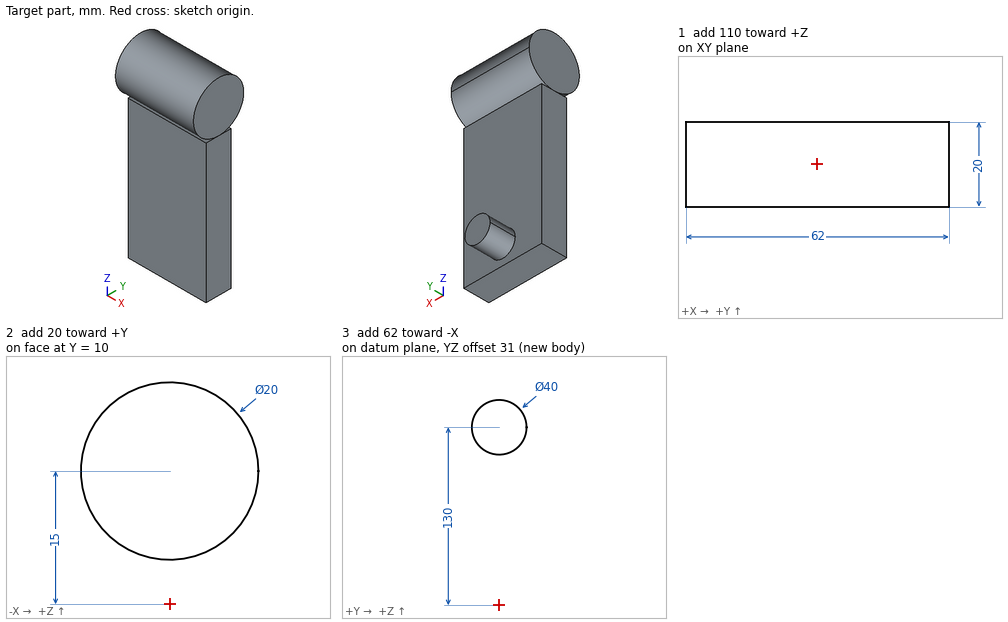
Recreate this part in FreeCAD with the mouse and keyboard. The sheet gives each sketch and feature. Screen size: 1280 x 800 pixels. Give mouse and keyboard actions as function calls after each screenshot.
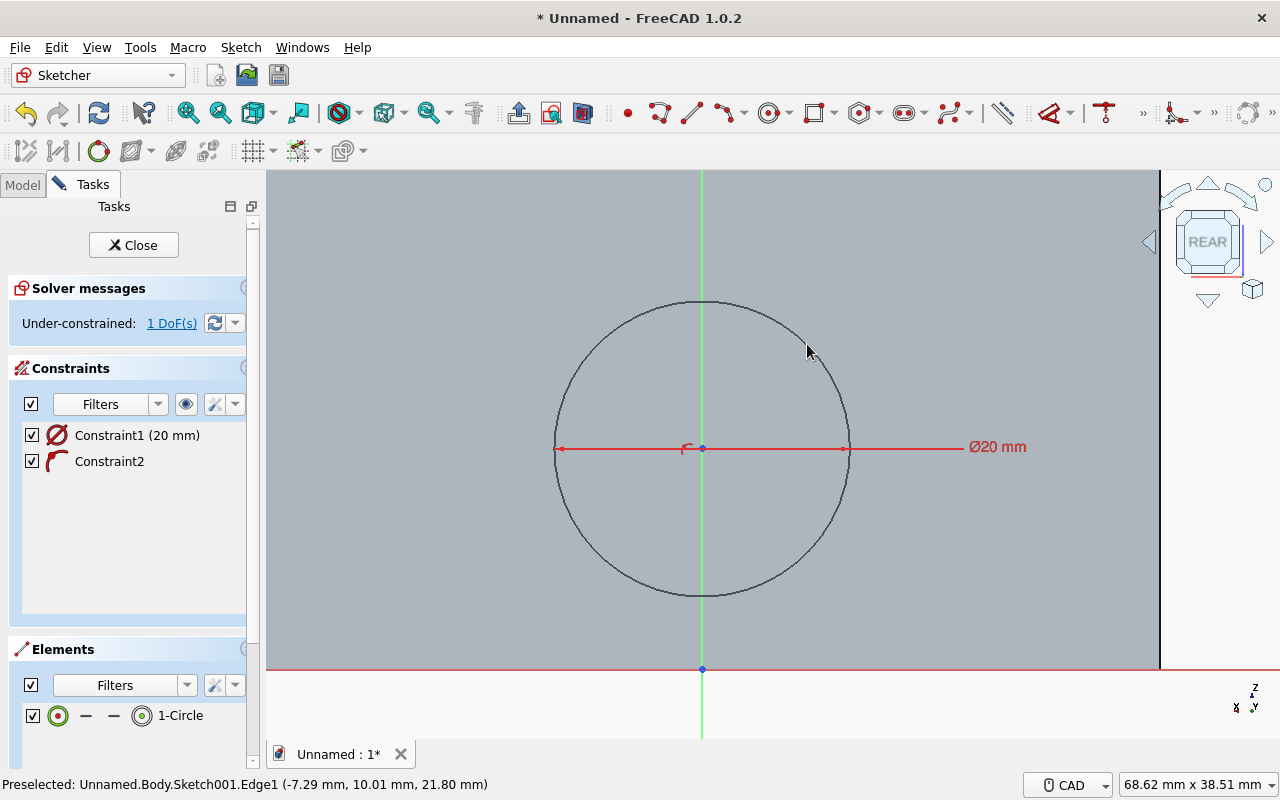
key(d)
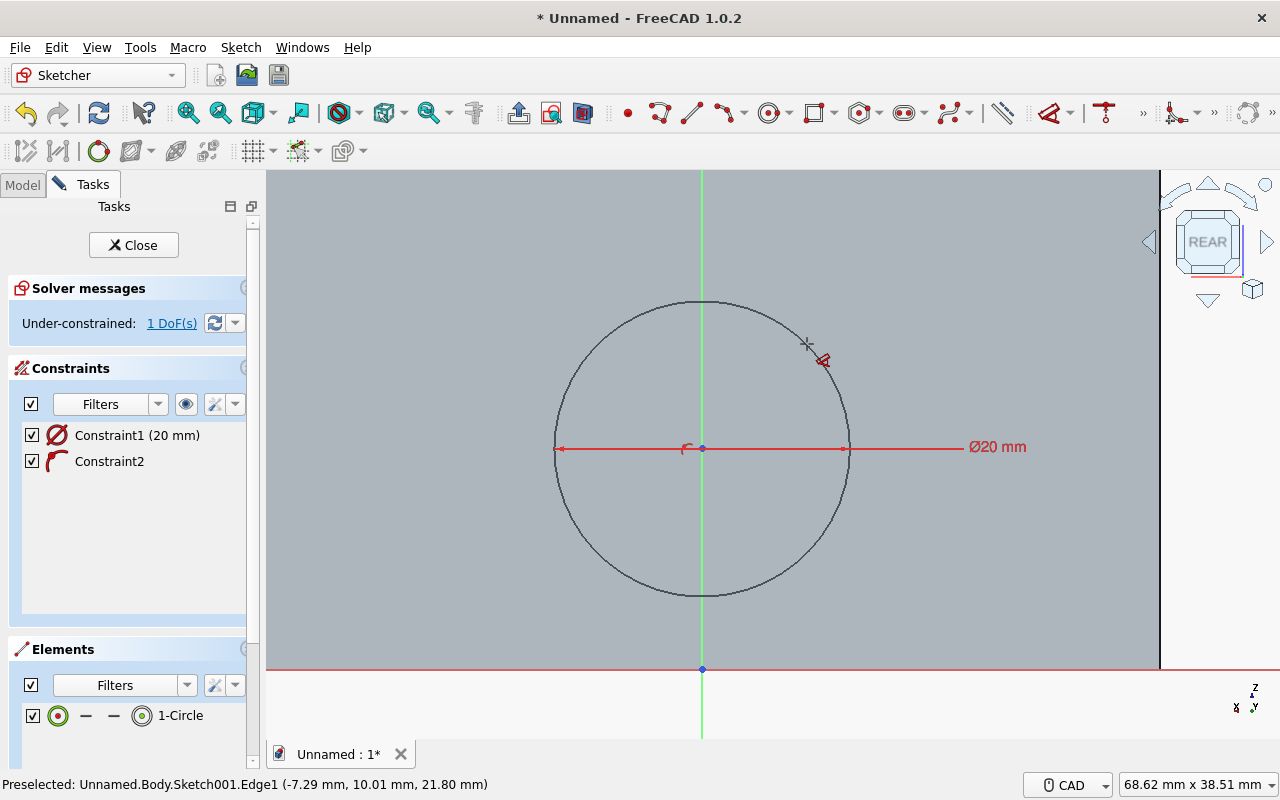
click(702, 449)
click(736, 559)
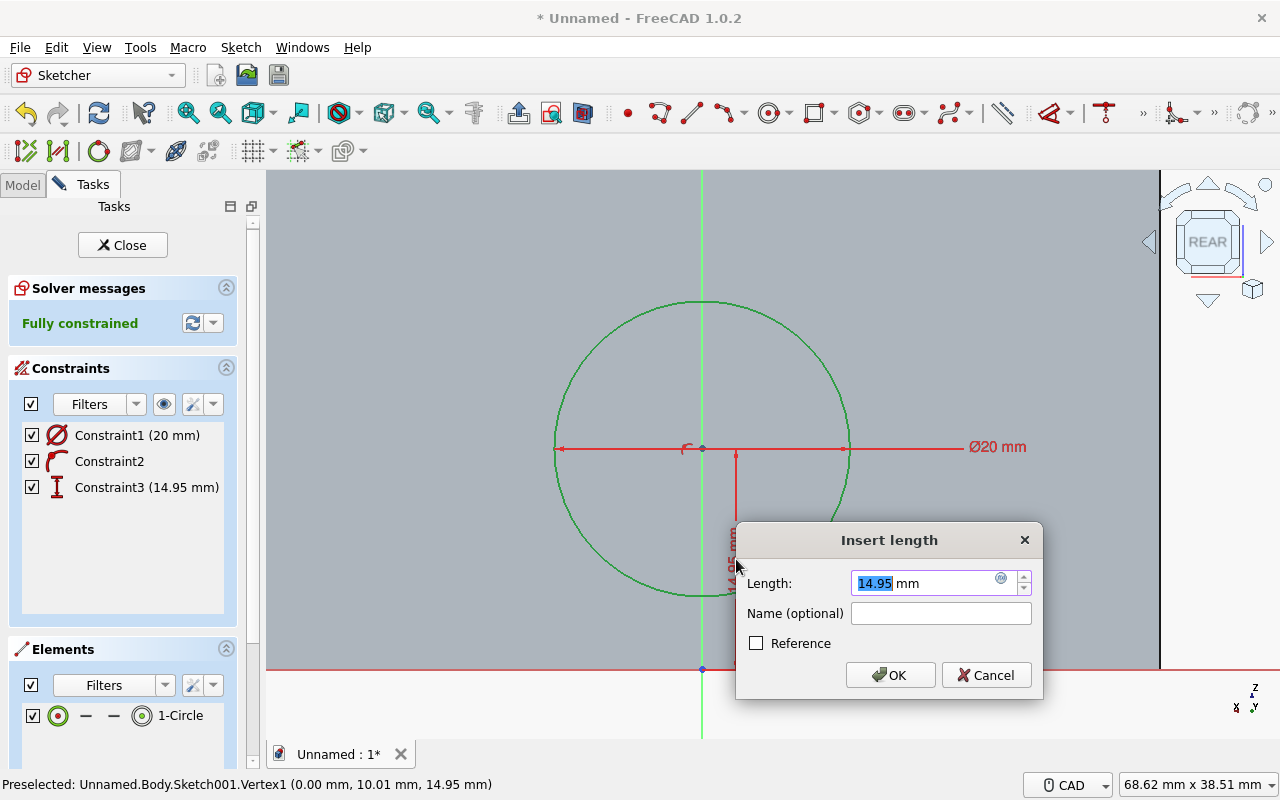
text(15)
key(Return)
key(Escape)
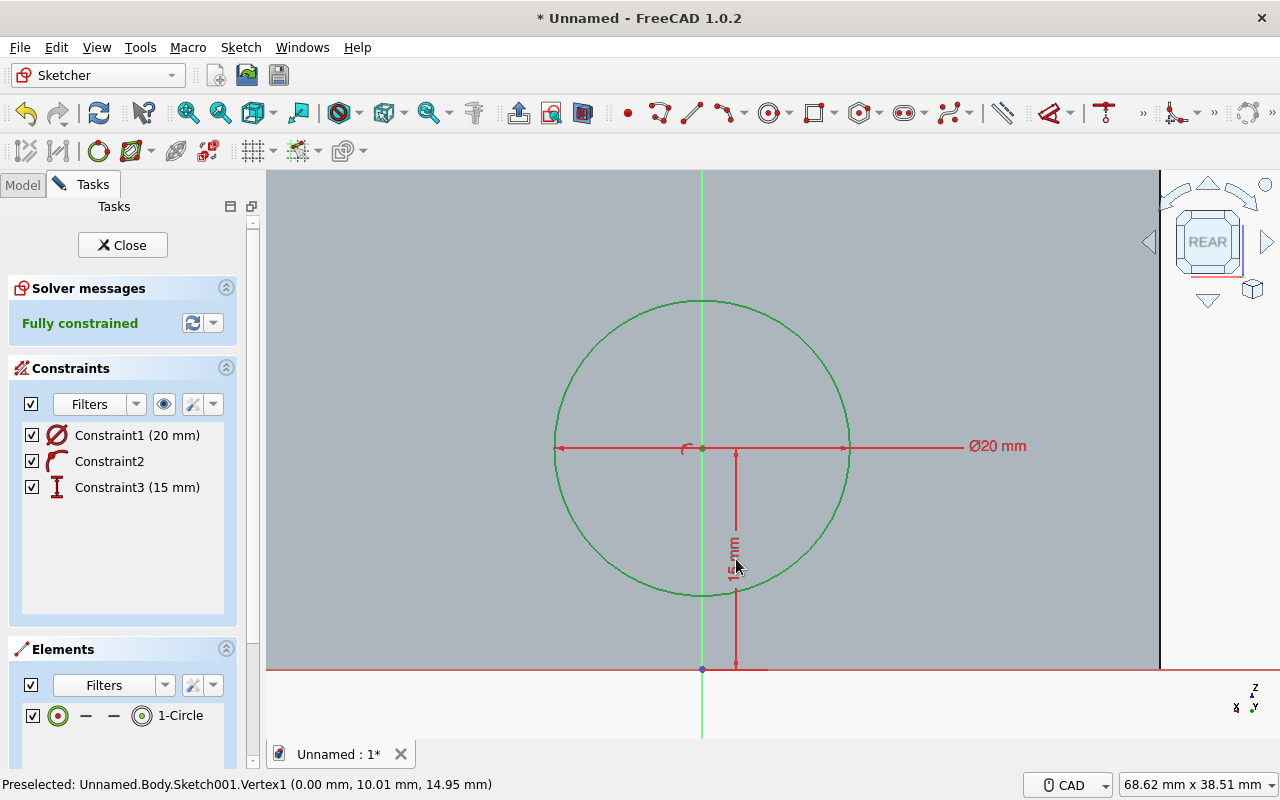
click(123, 245)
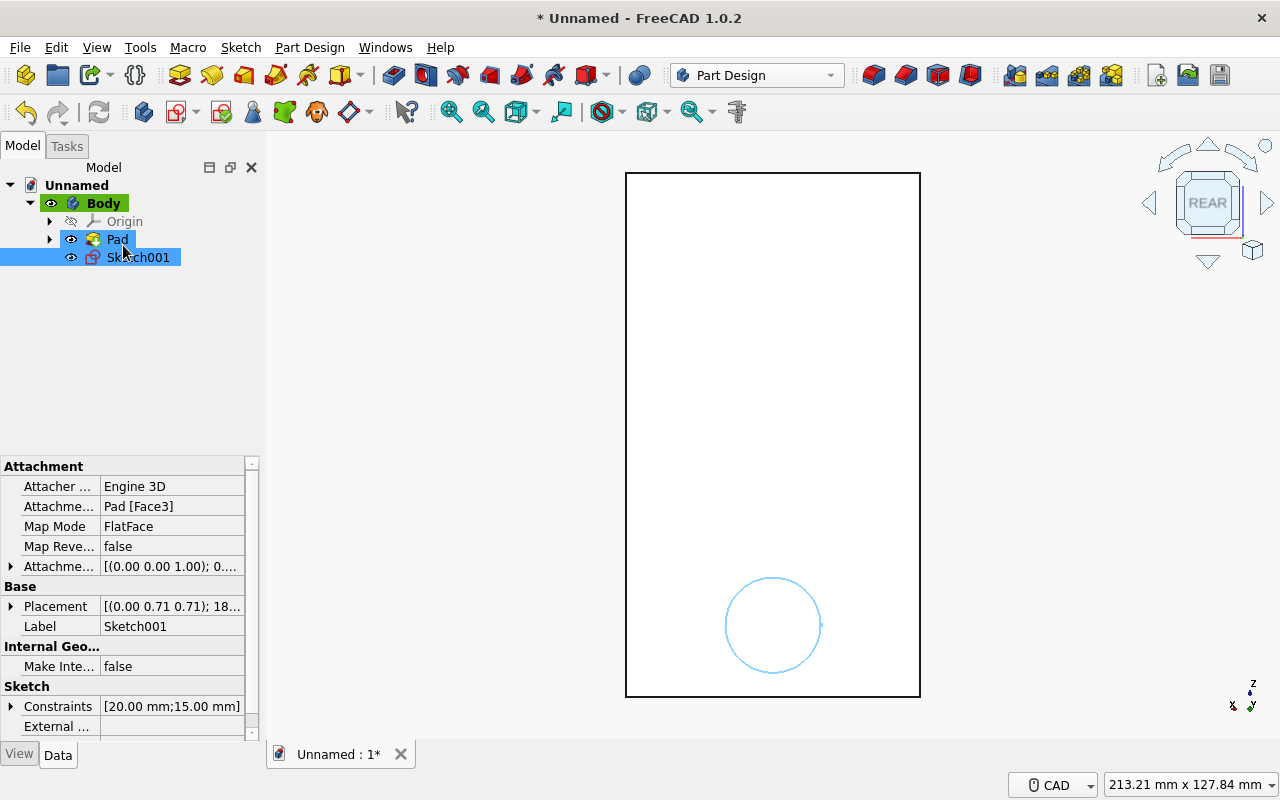
click(180, 76)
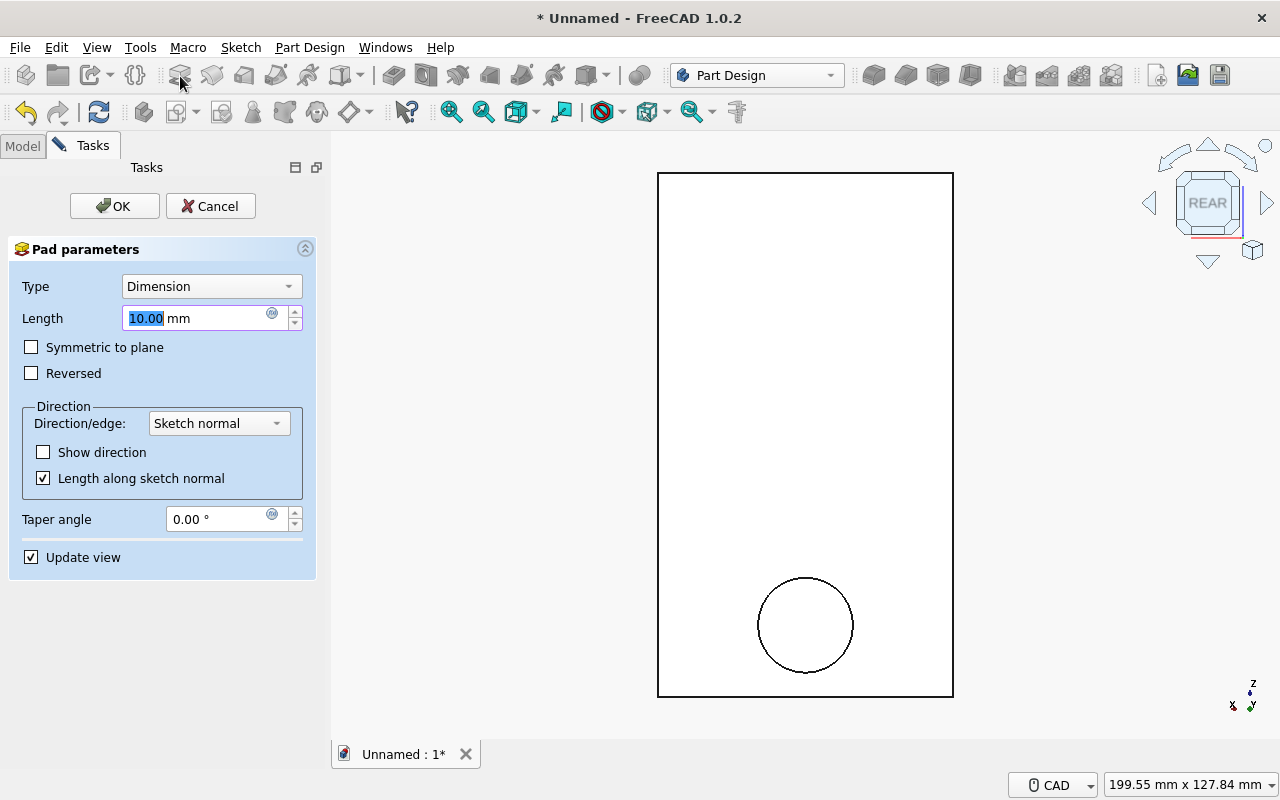
text(20)
key(Tab)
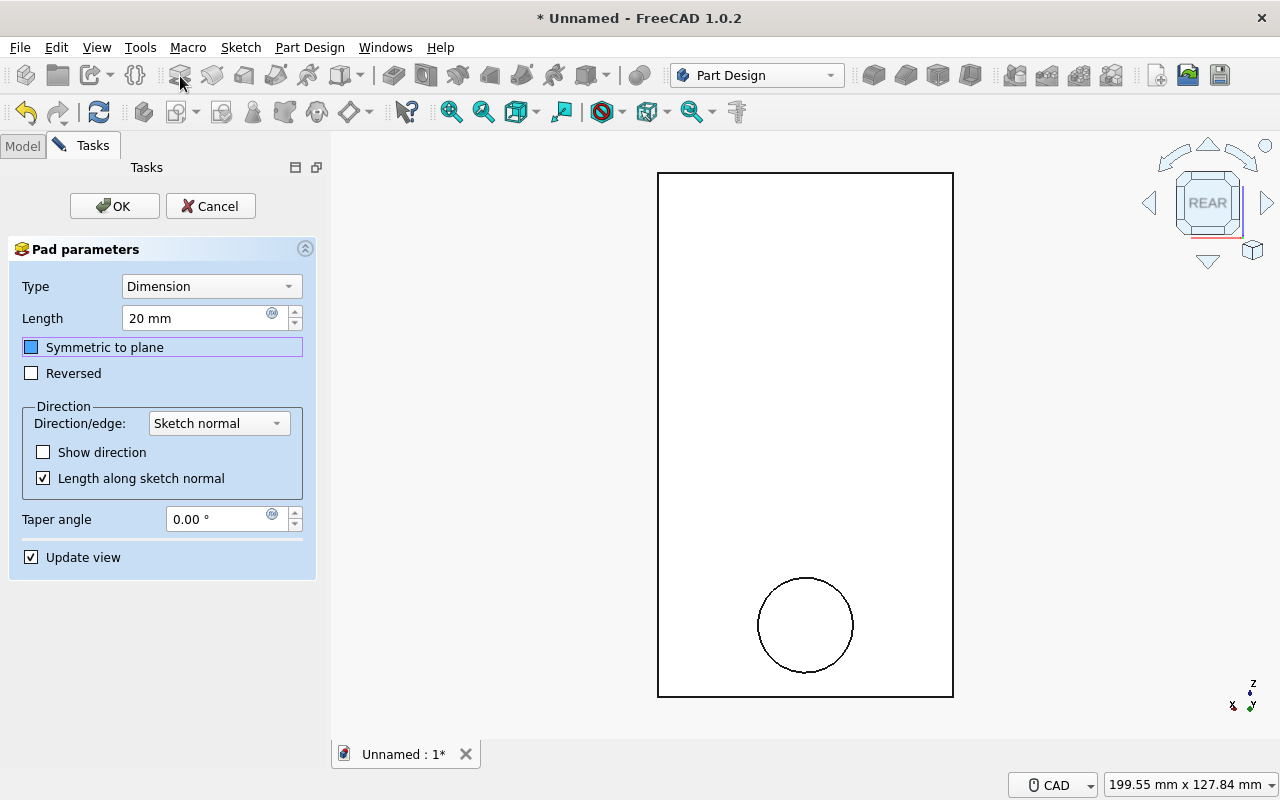
click(115, 206)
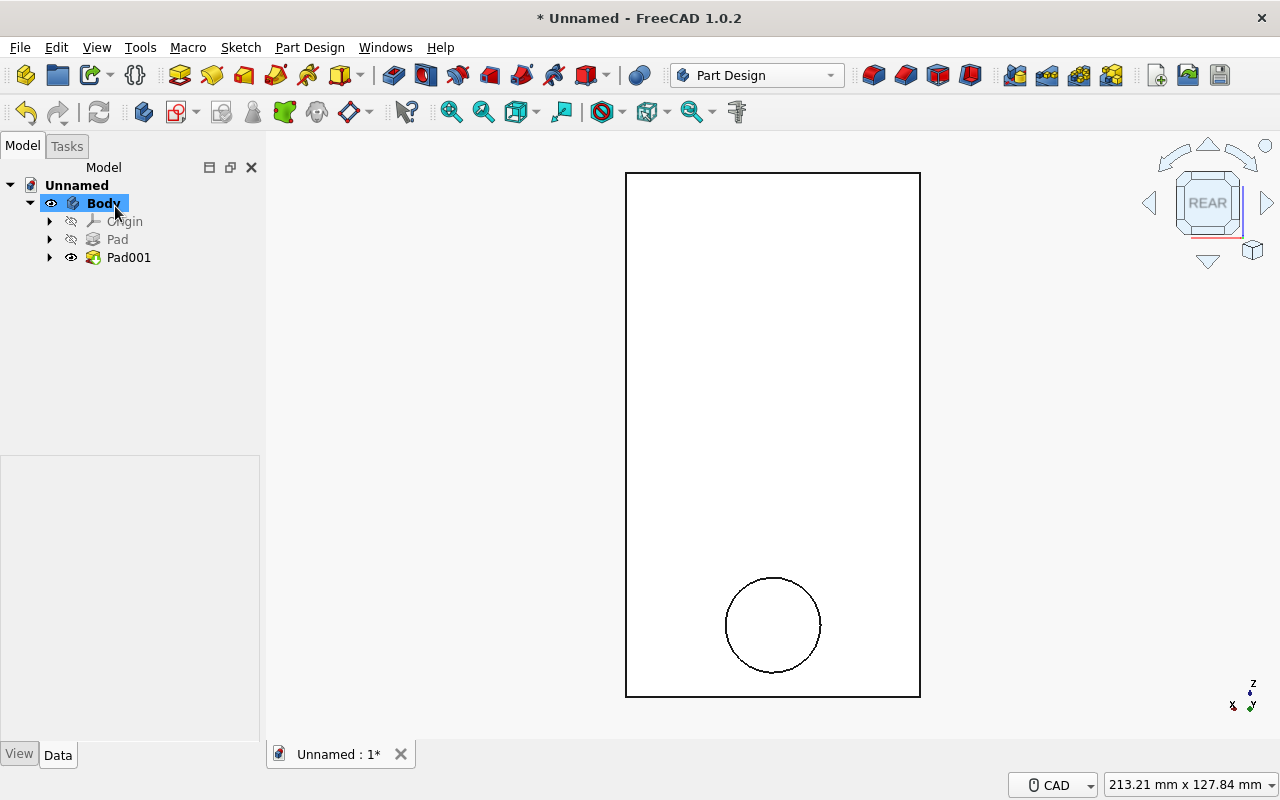
click(144, 112)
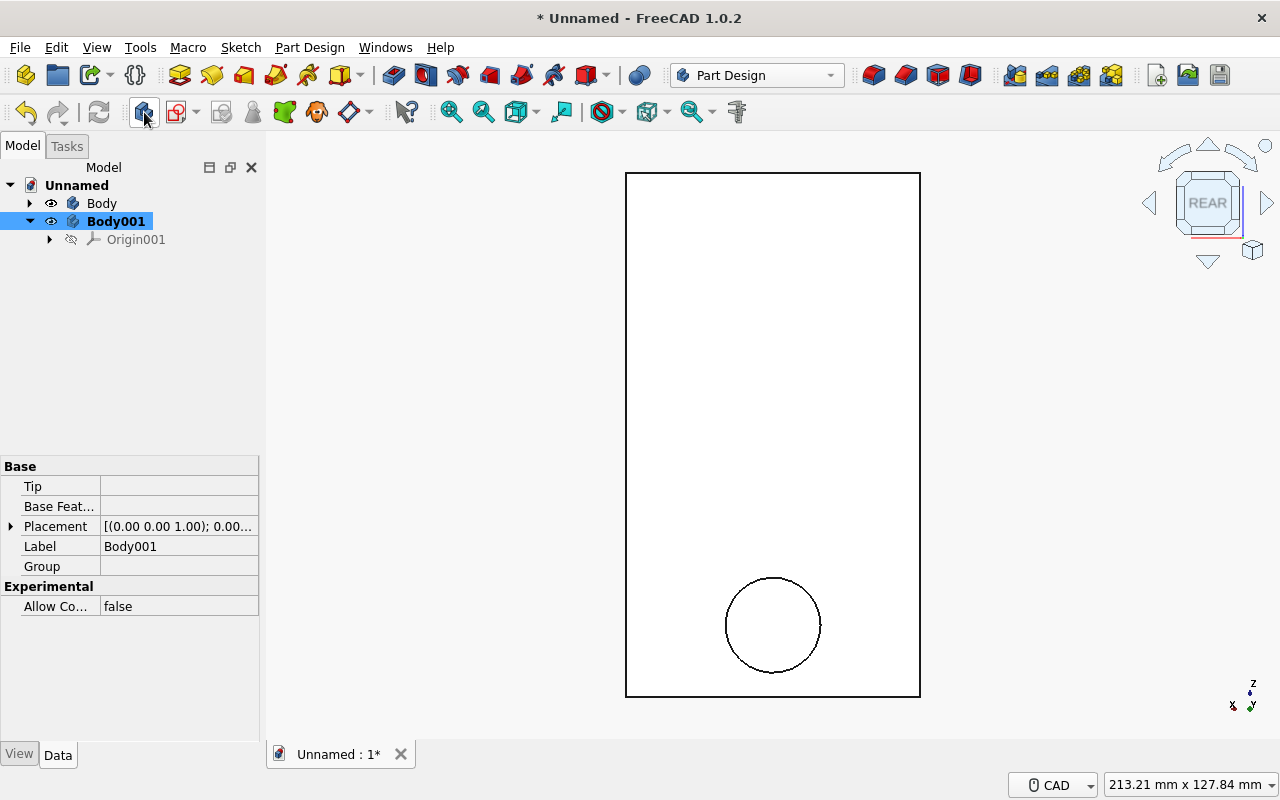
click(50, 239)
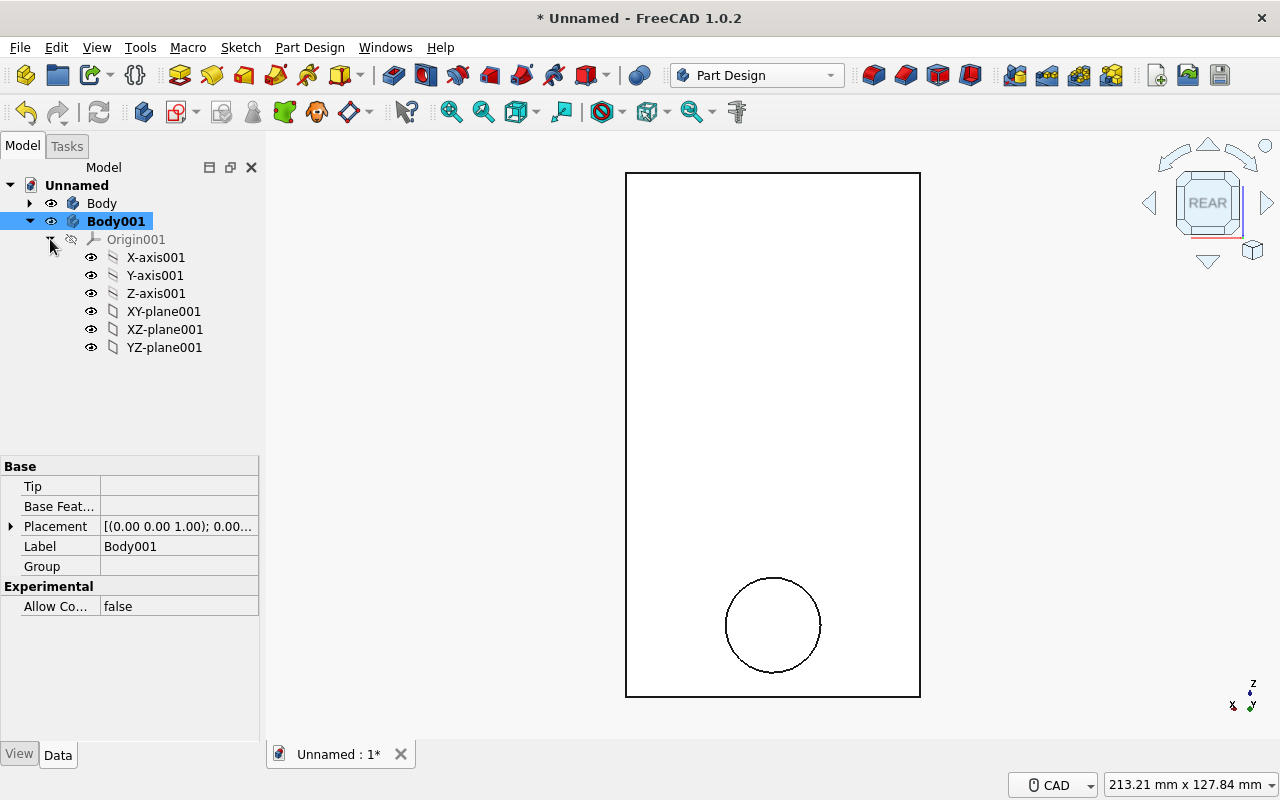
click(136, 347)